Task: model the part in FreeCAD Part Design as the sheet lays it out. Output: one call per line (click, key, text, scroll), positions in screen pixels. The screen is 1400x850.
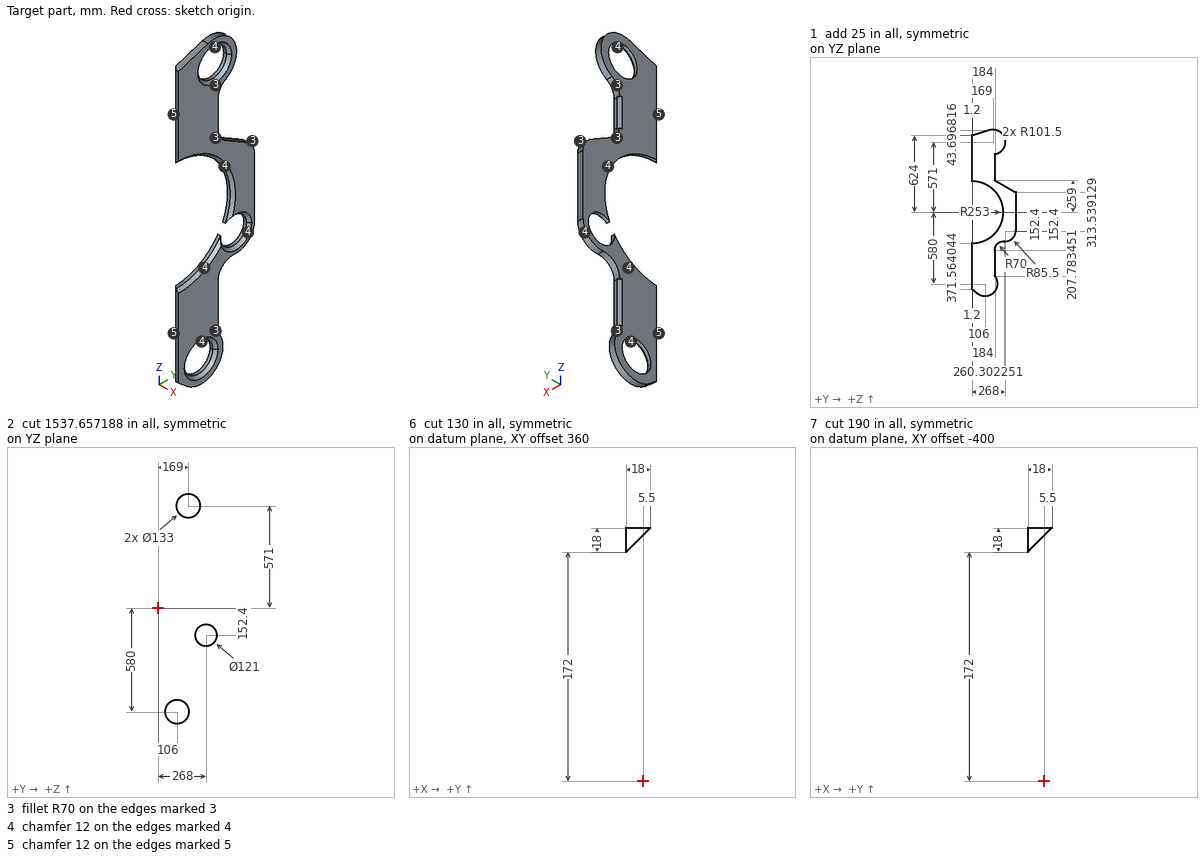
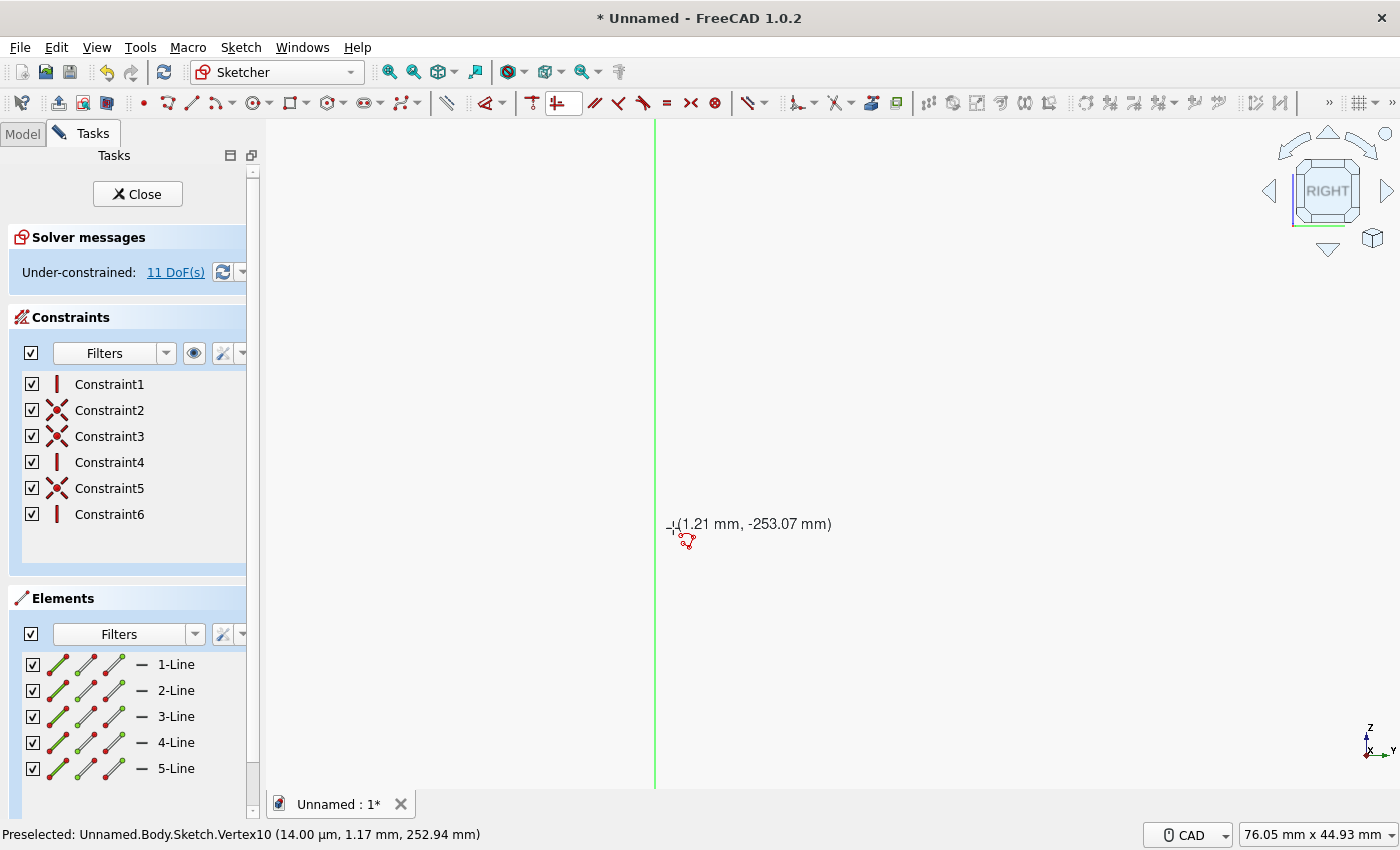
scroll(694, 560, down, 18)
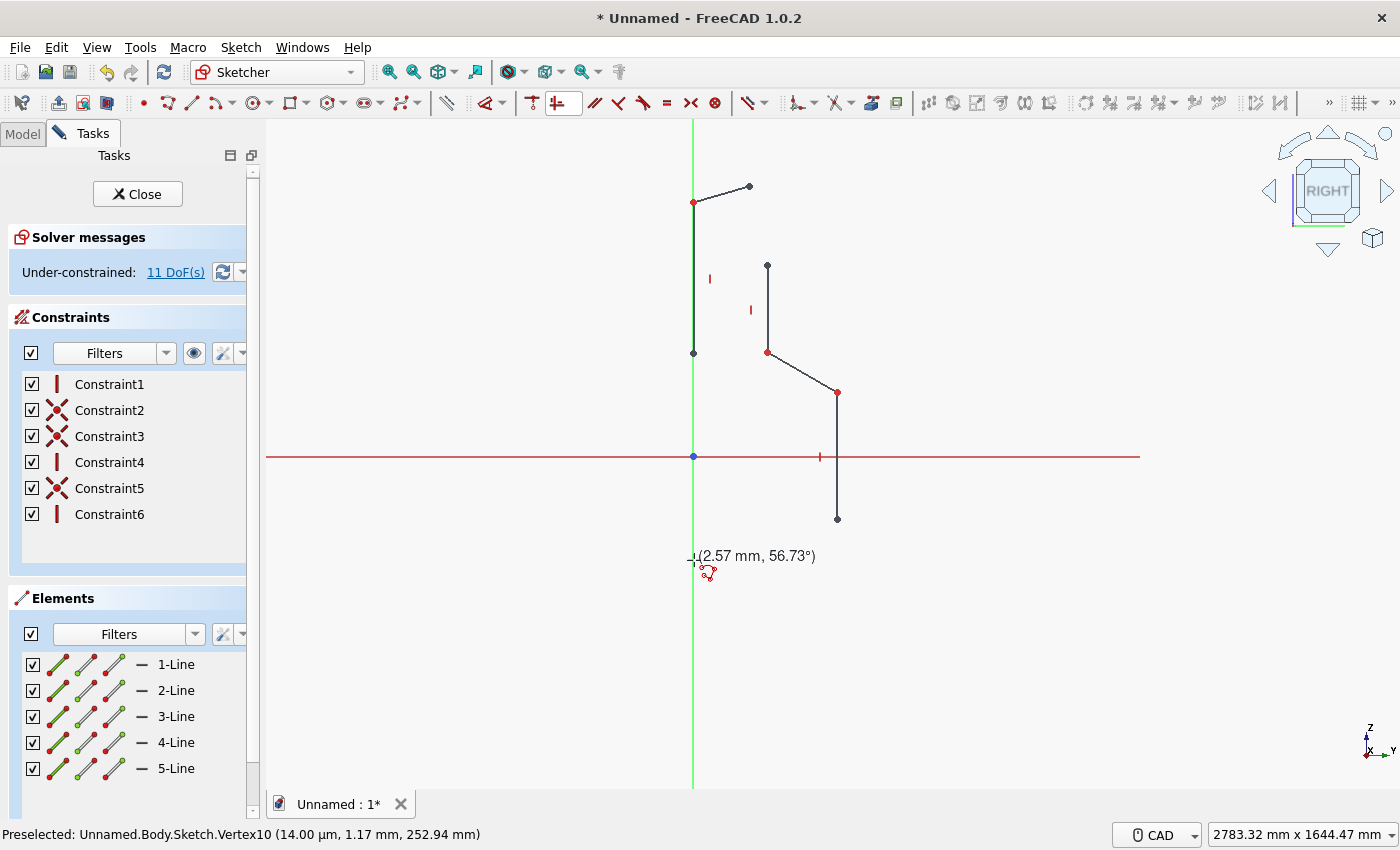
scroll(694, 711, up, 18)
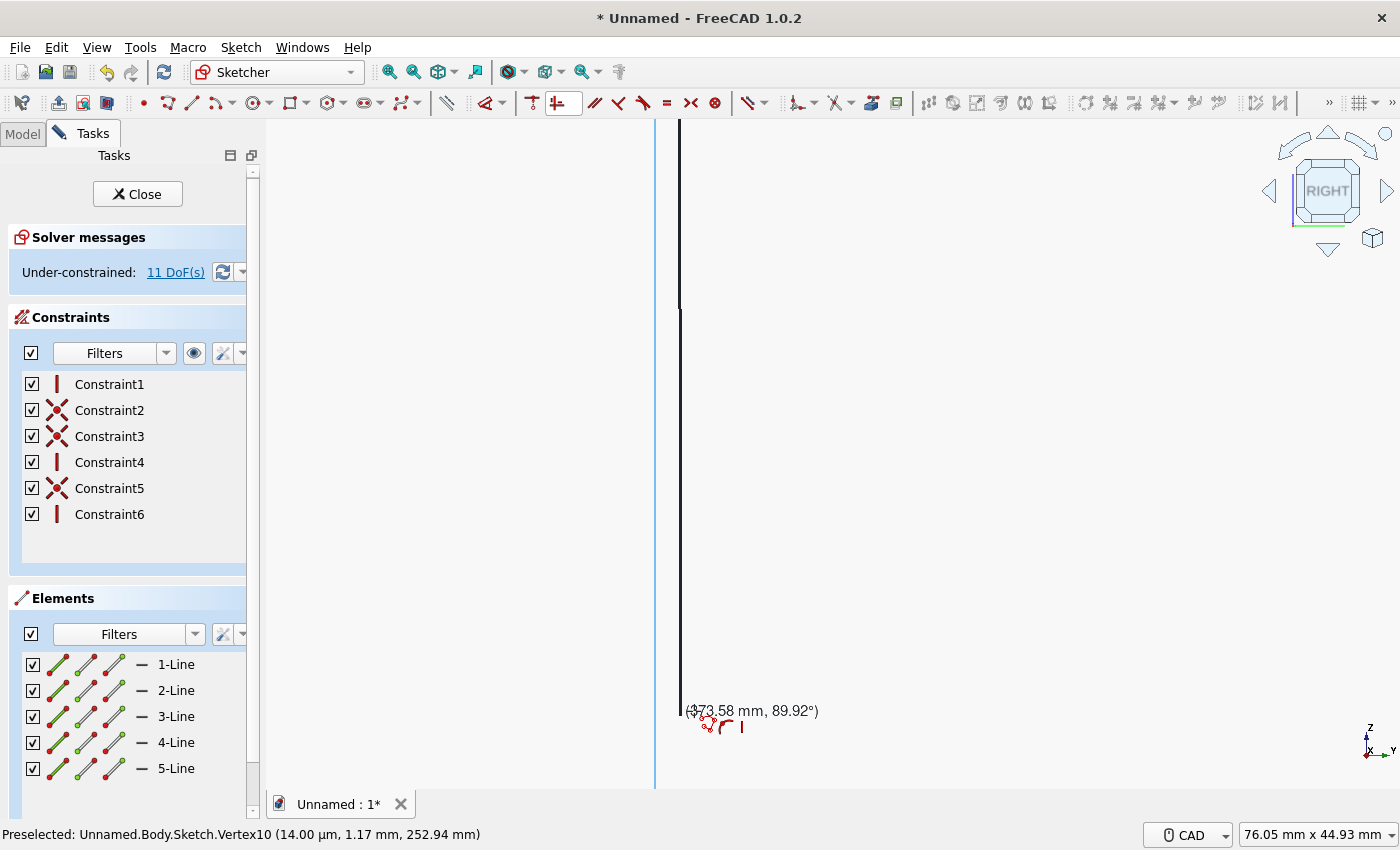
click(673, 685)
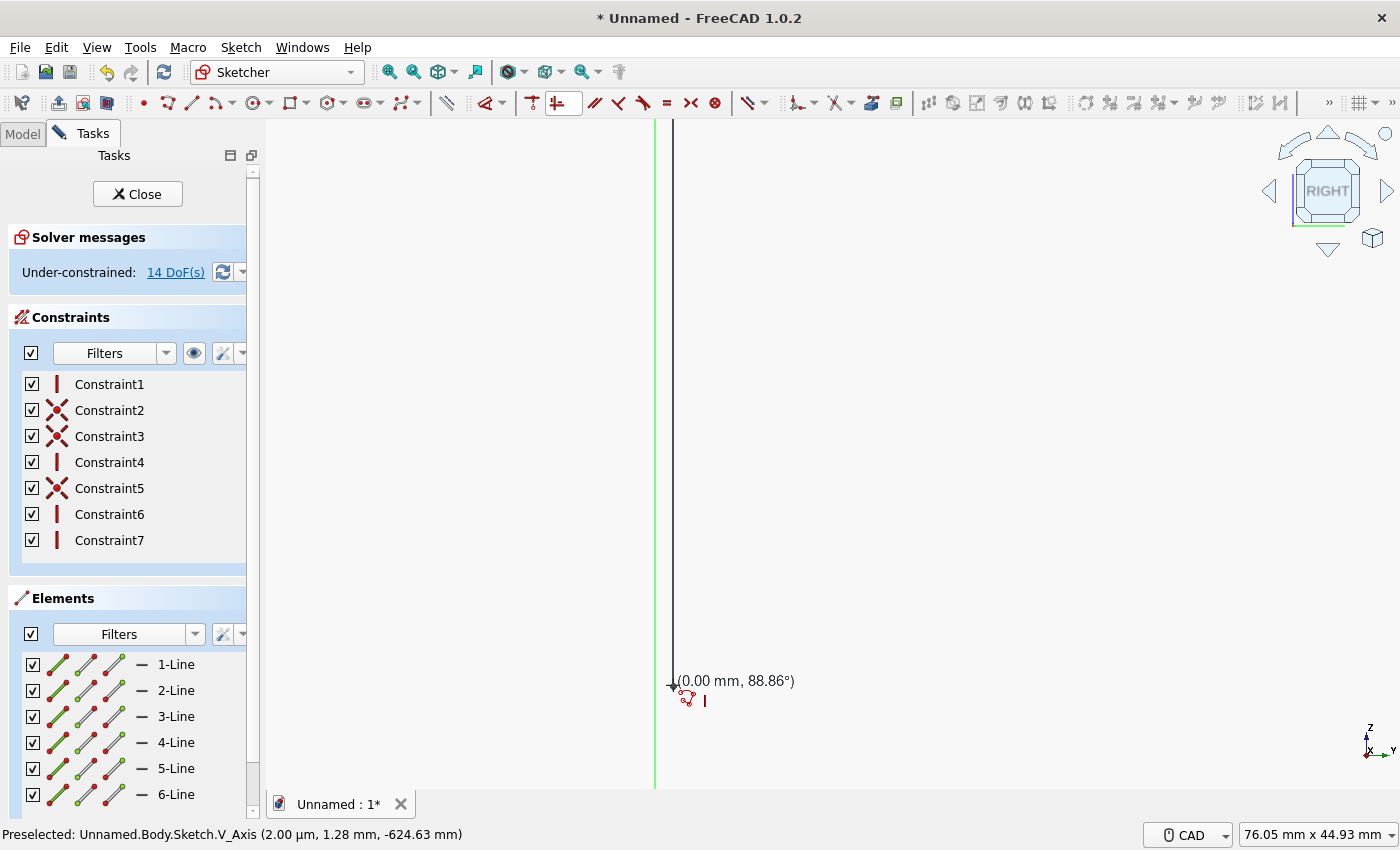
scroll(694, 711, down, 18)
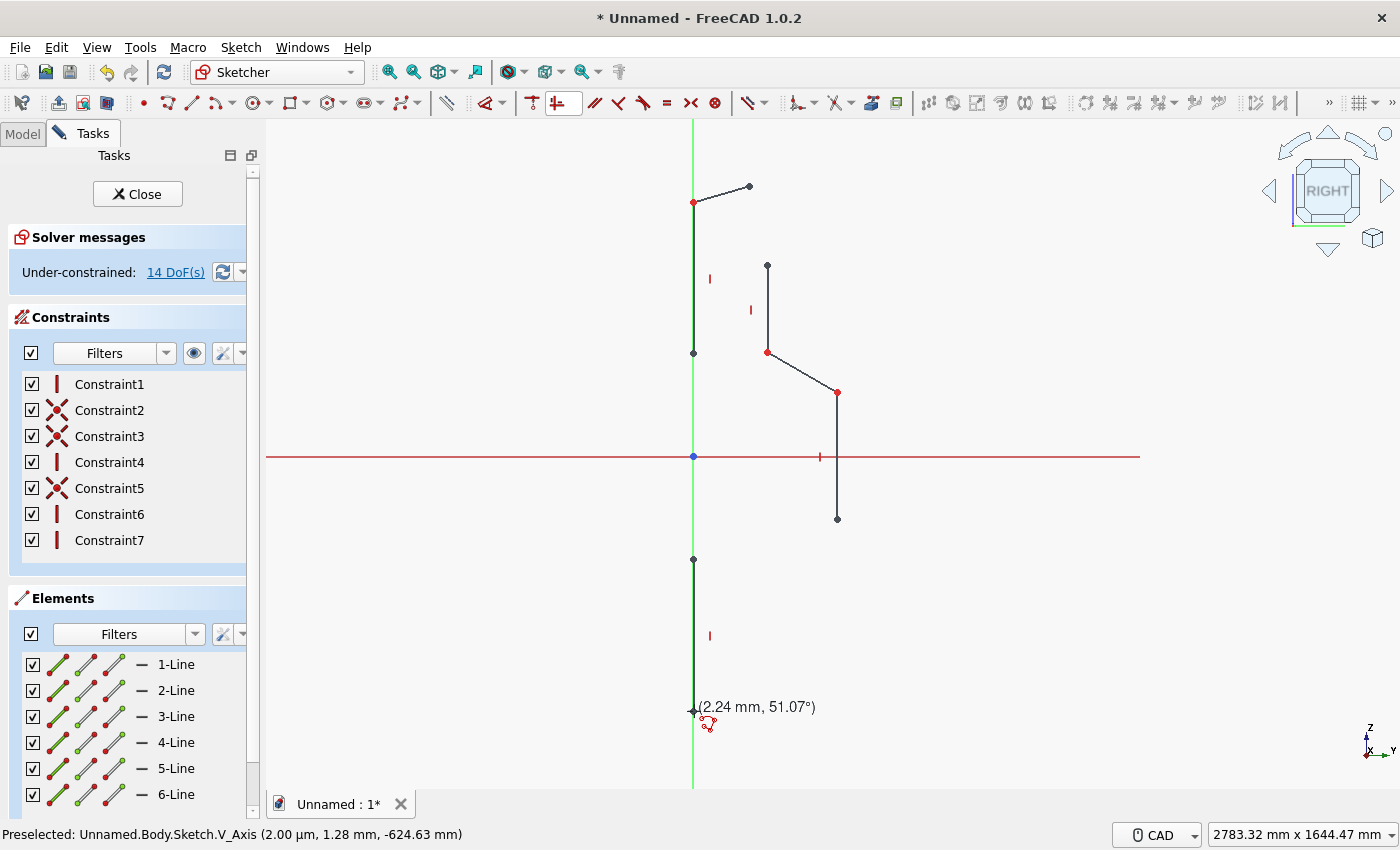
click(710, 725)
right_click(710, 725)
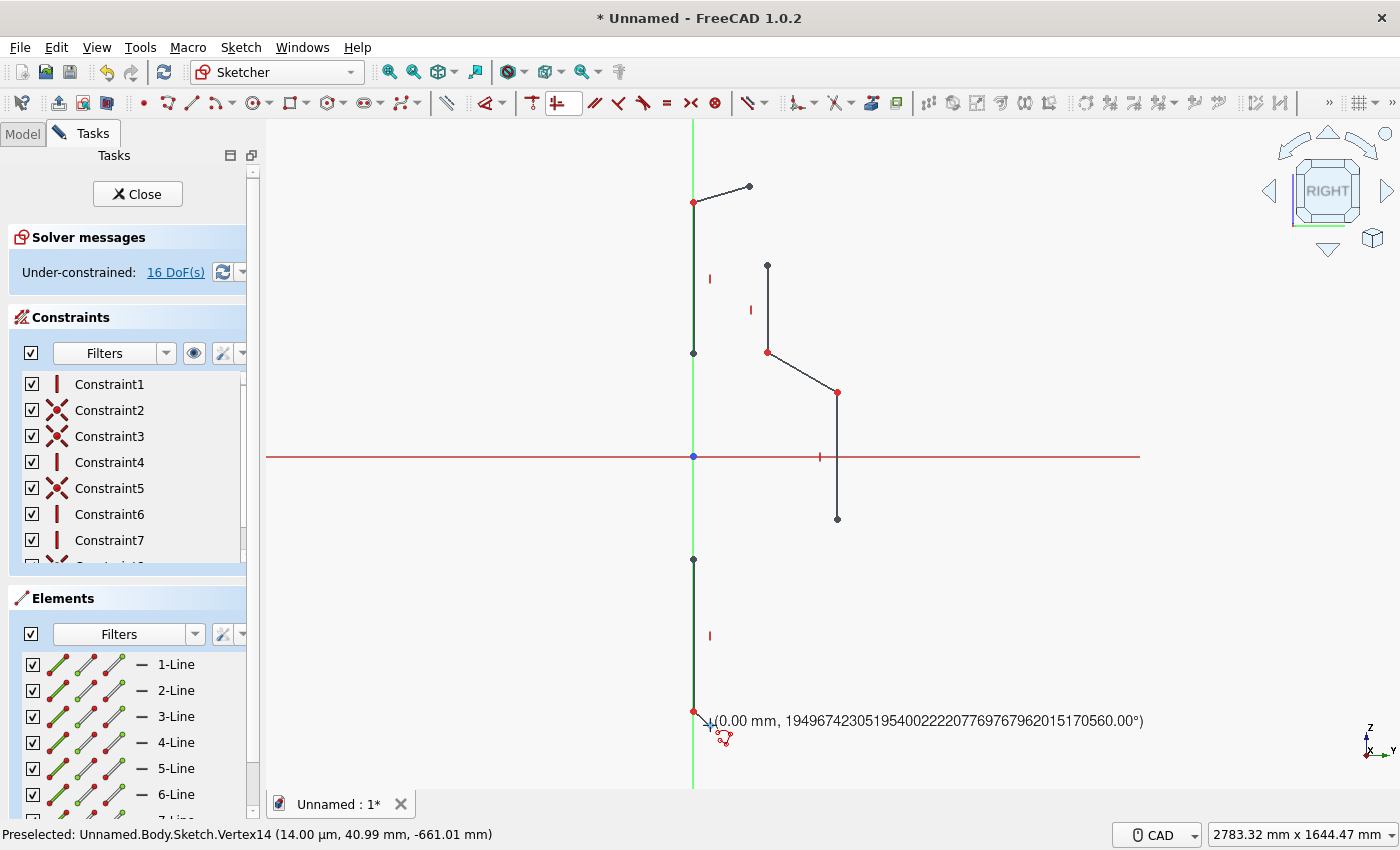
key(g)
key(l)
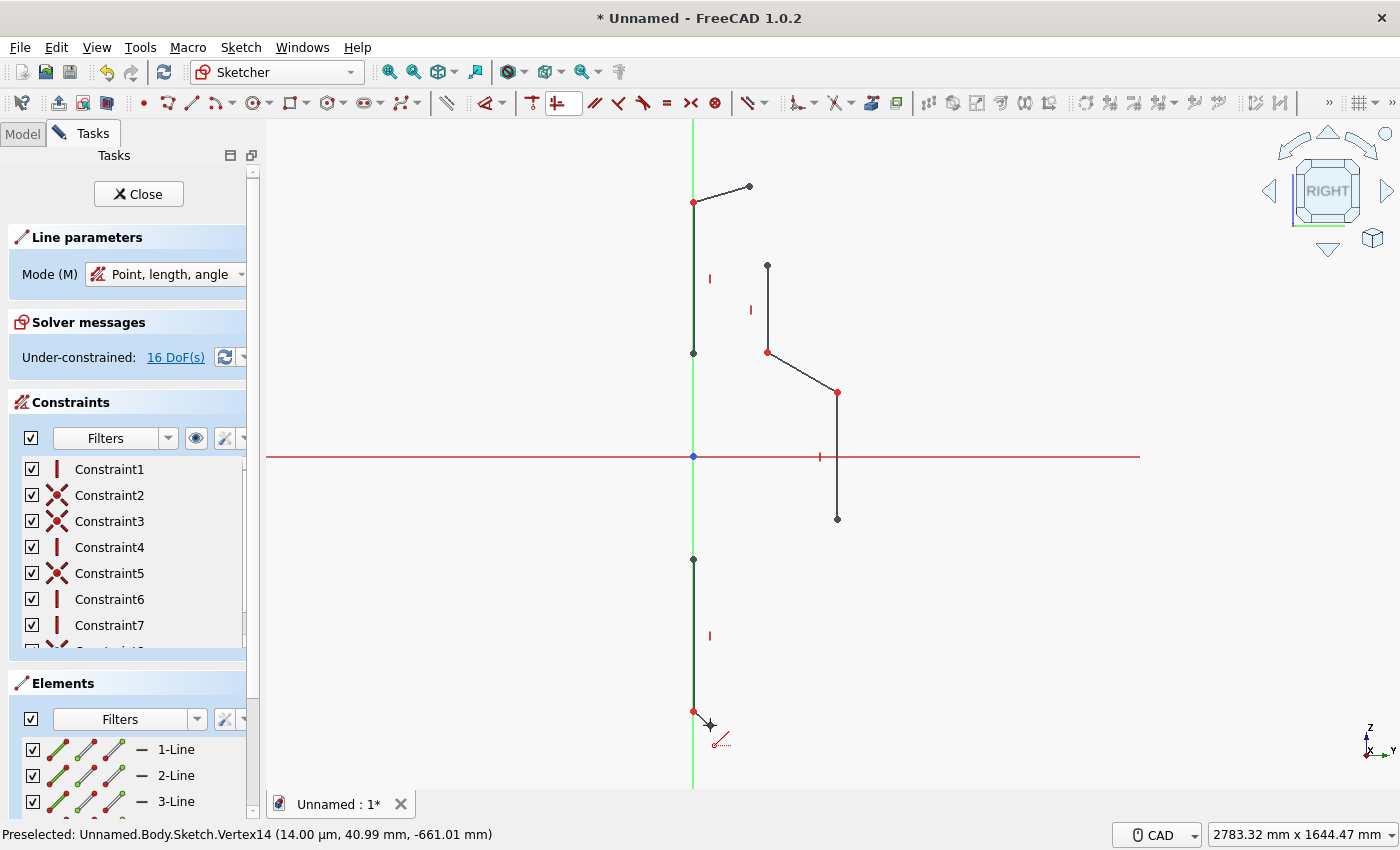
click(768, 667)
click(768, 582)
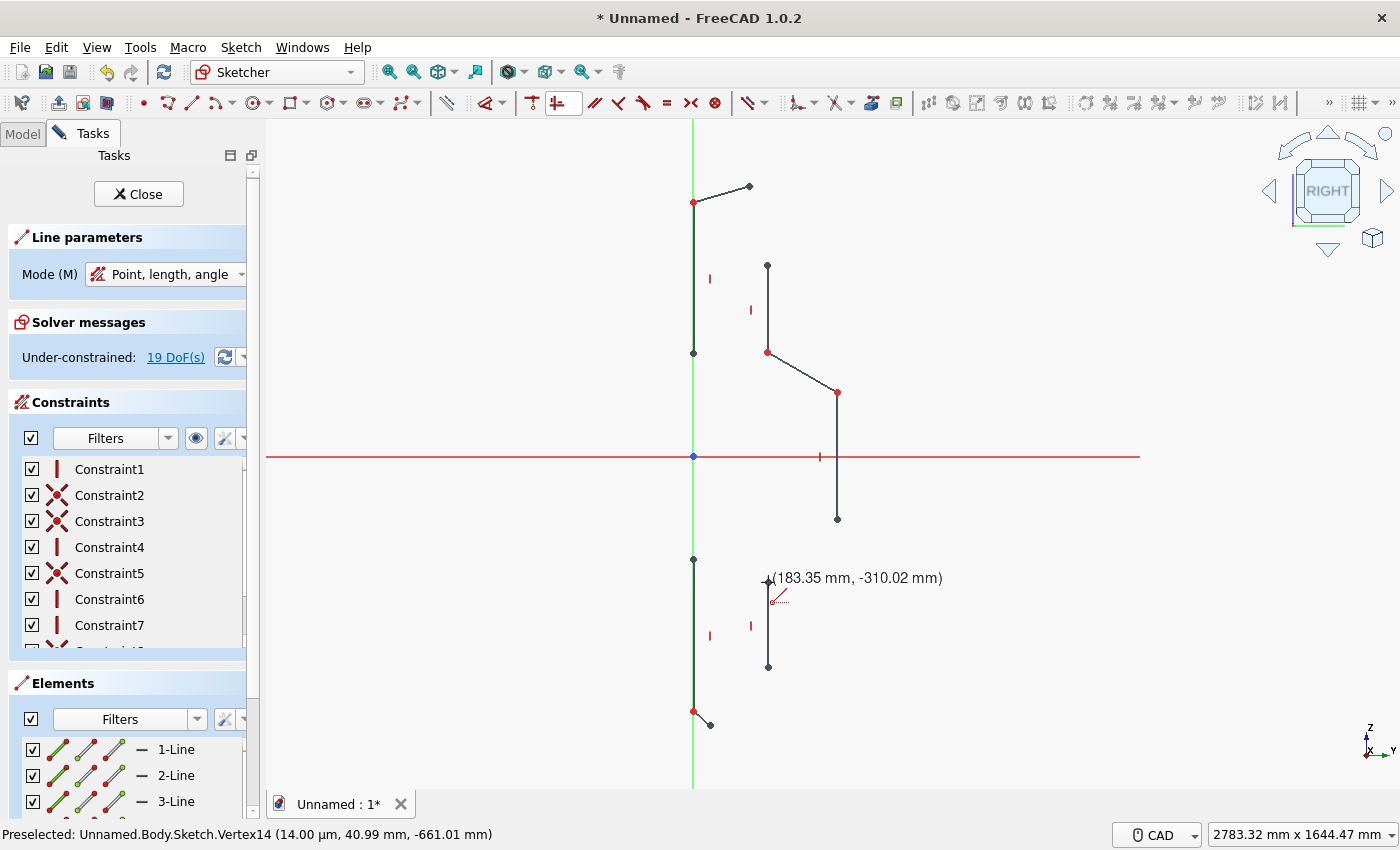
key(g)
key(3)
key(a)